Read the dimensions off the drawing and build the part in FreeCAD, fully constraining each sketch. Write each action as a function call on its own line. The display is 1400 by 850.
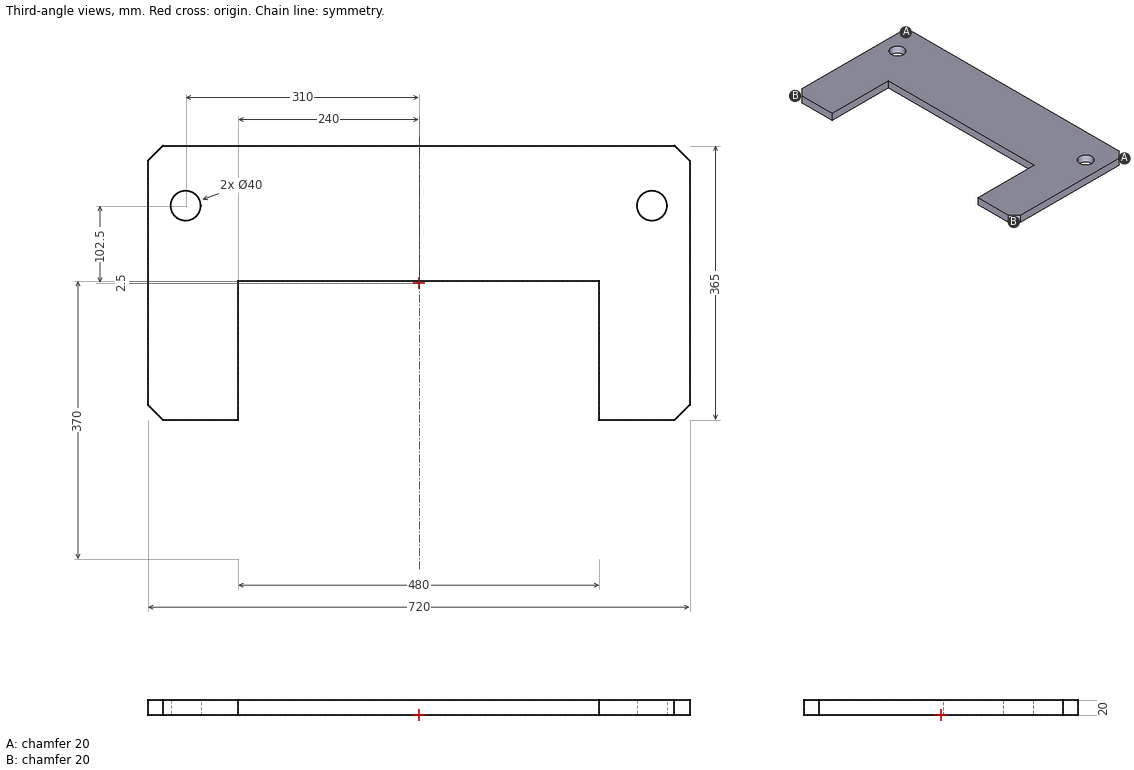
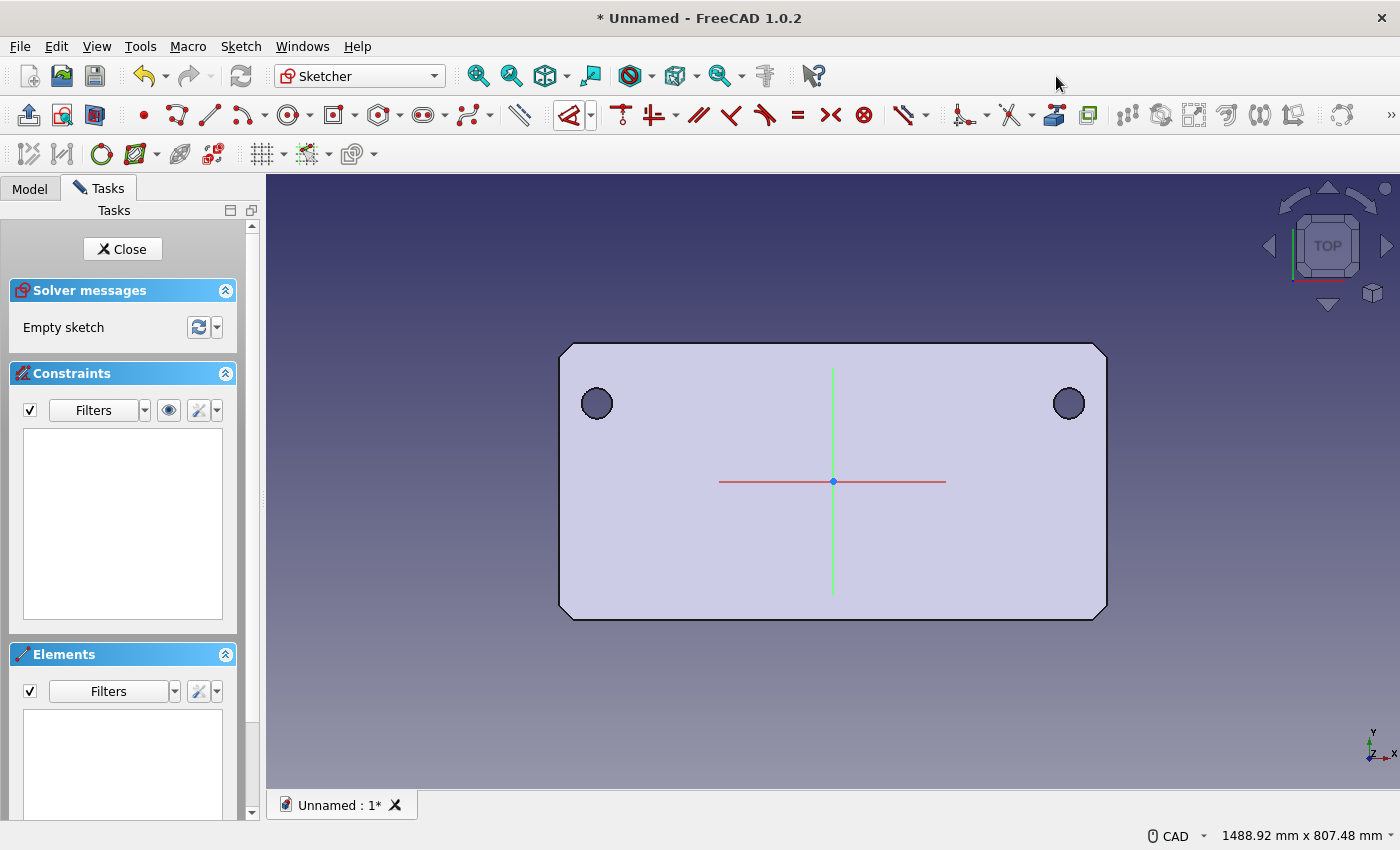
scroll(455, 202, down, 1)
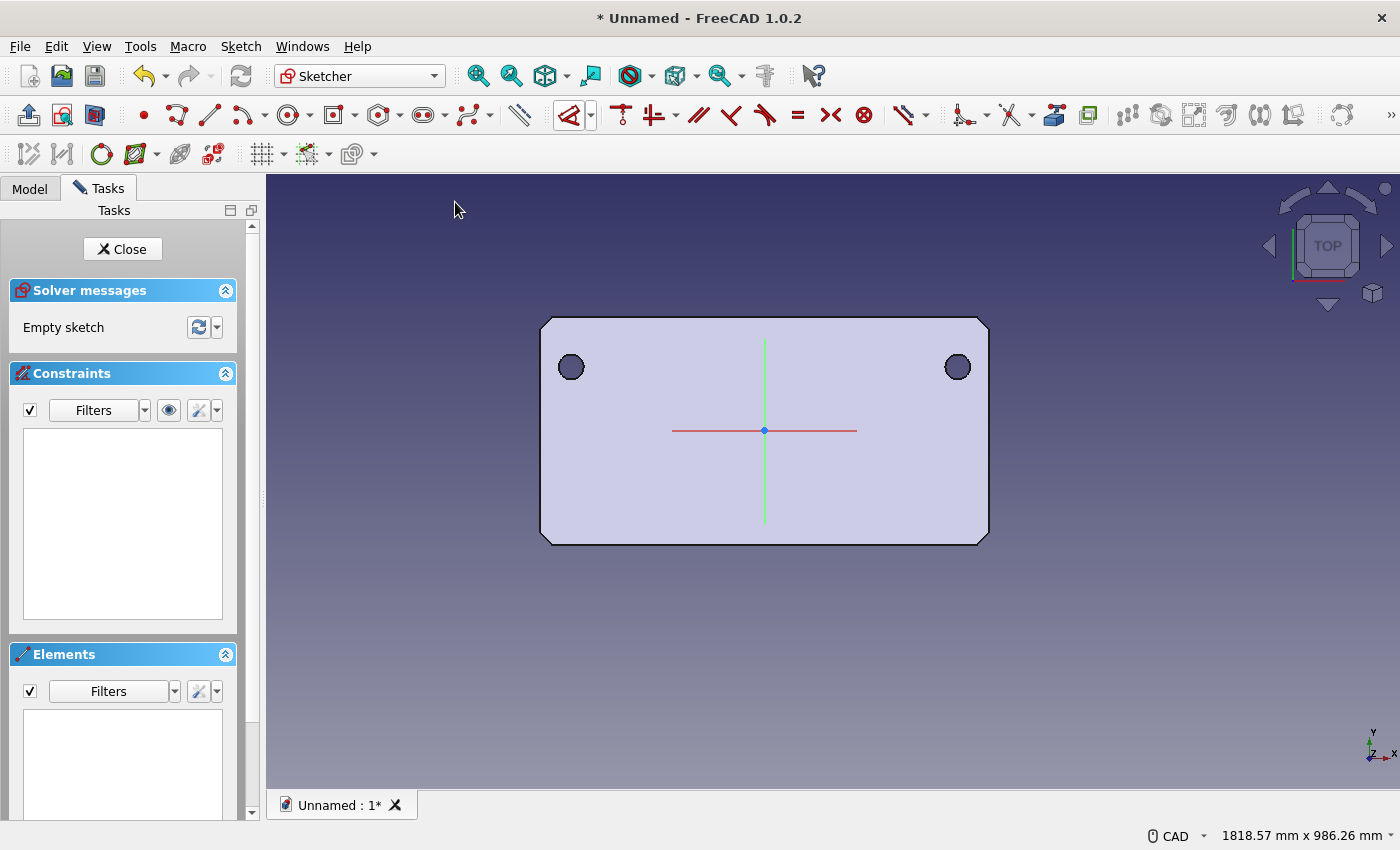
scroll(765, 621, up, 3)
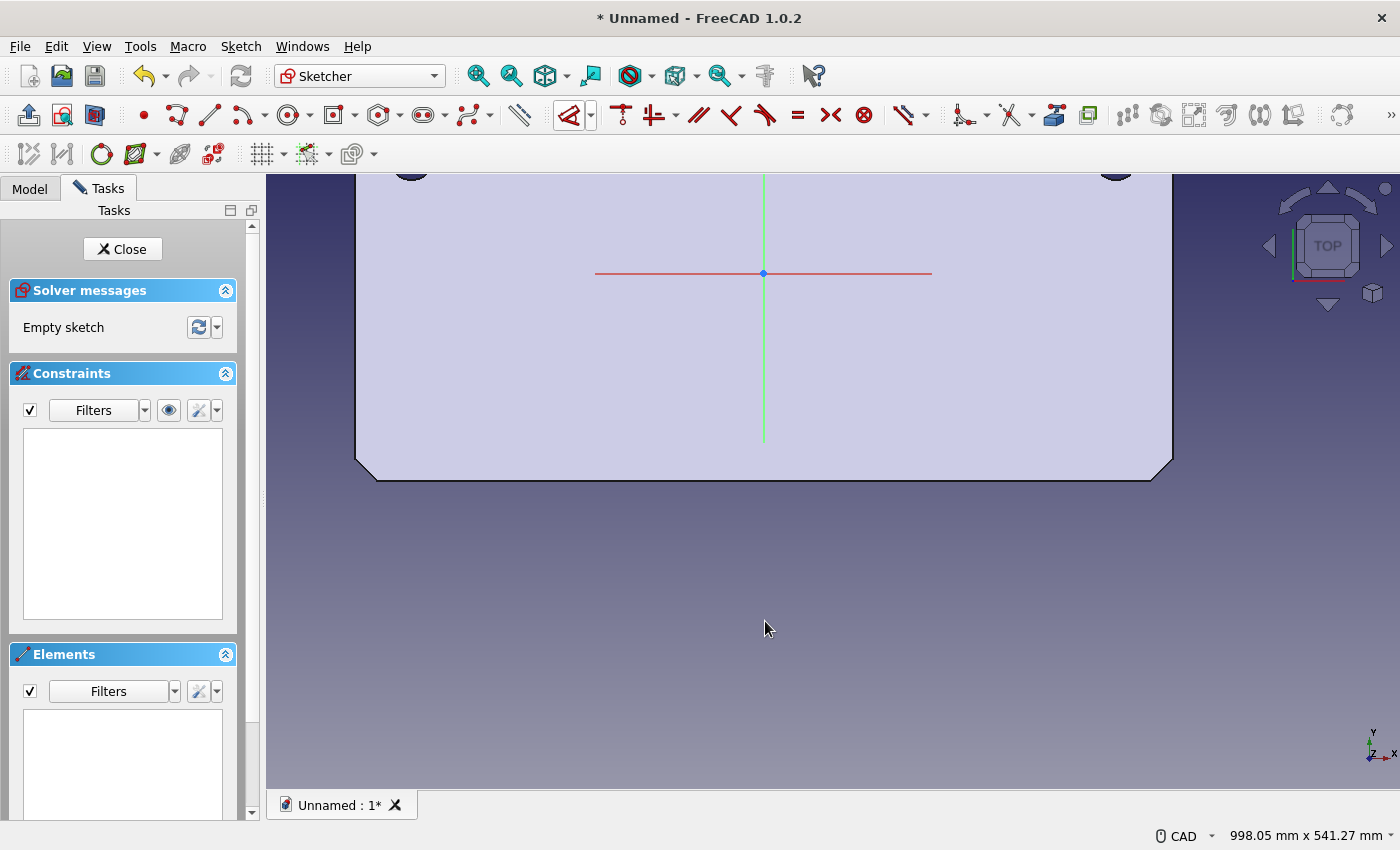
key(g)
key(r)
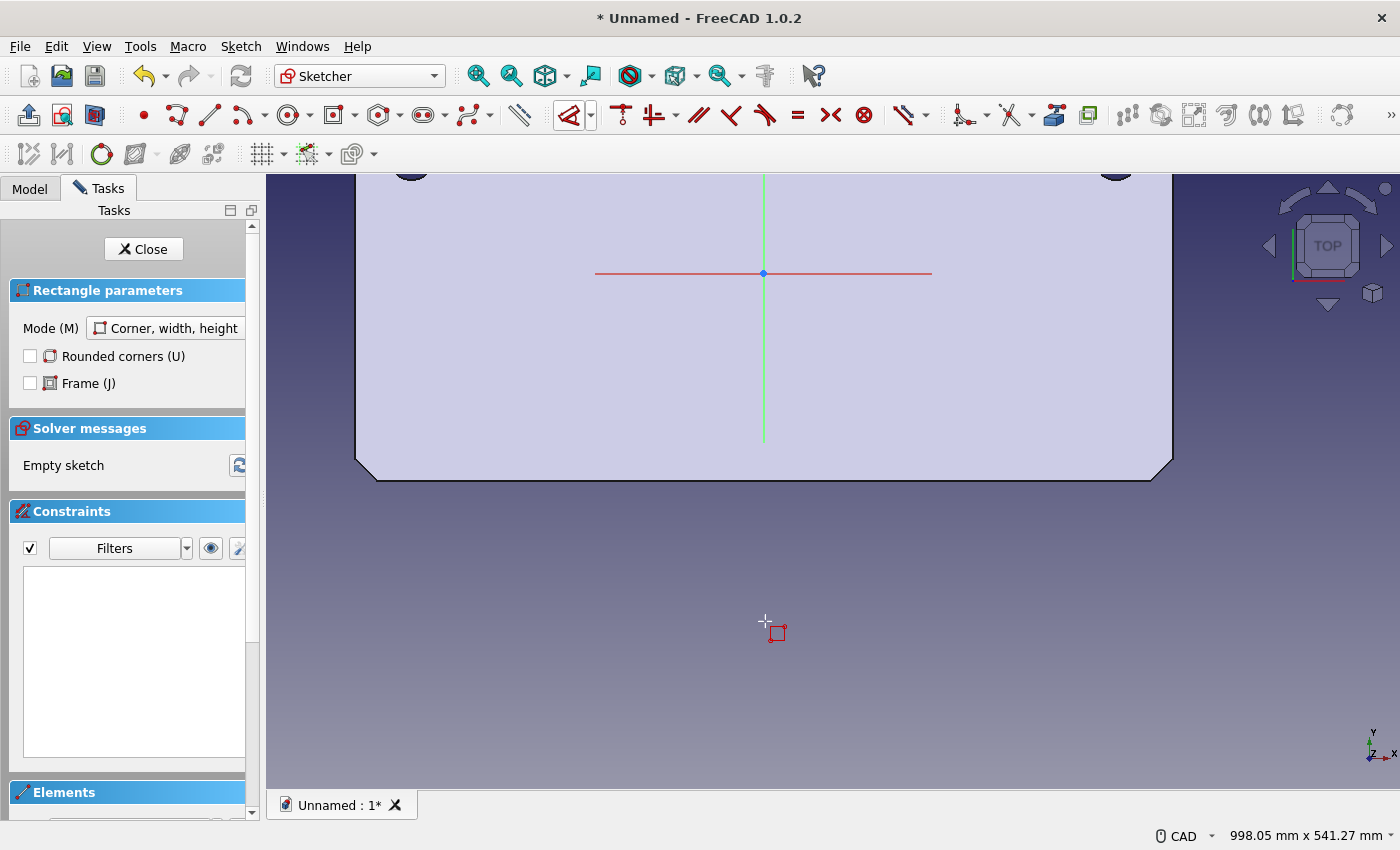
scroll(491, 271, up, 9)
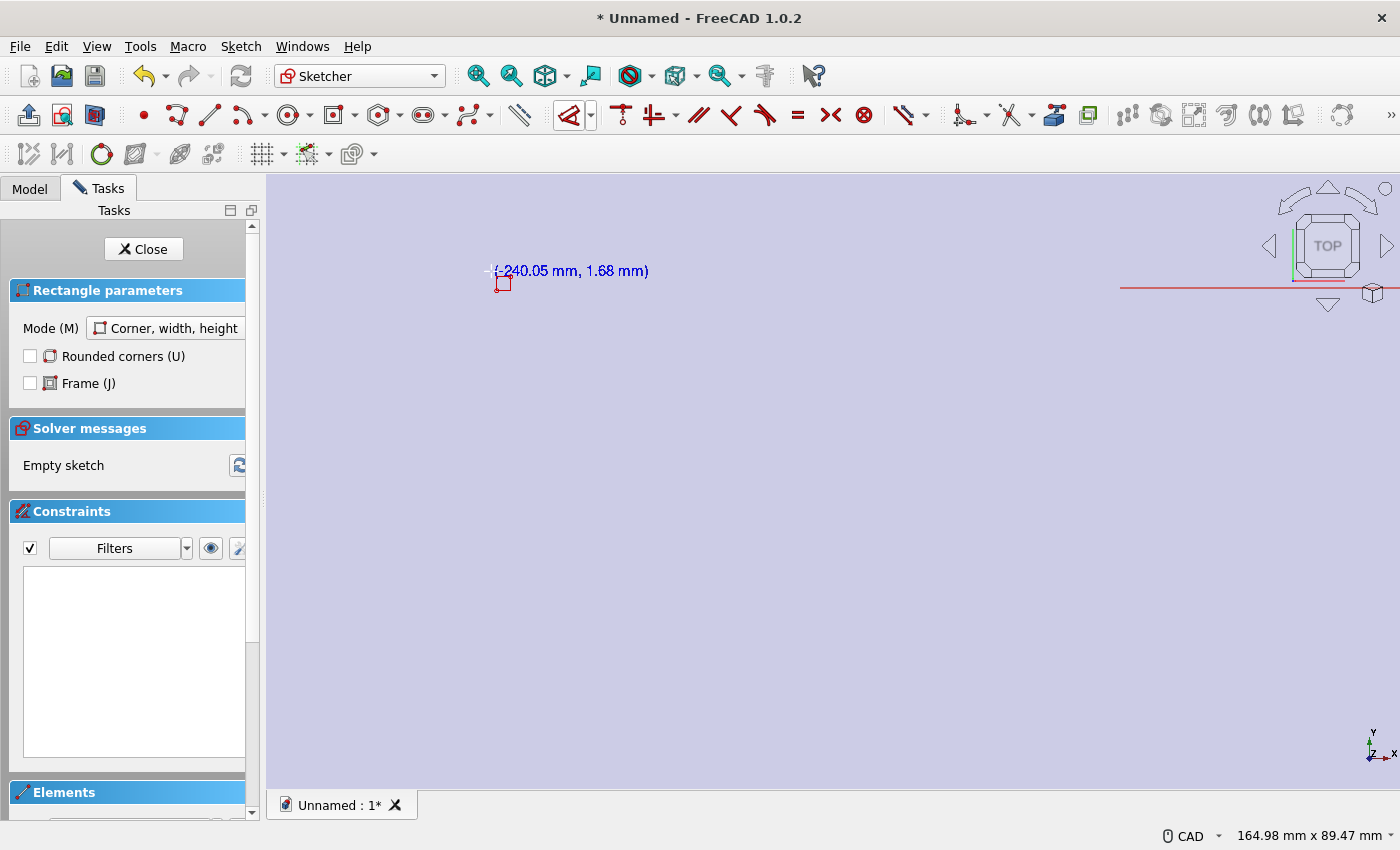
click(490, 271)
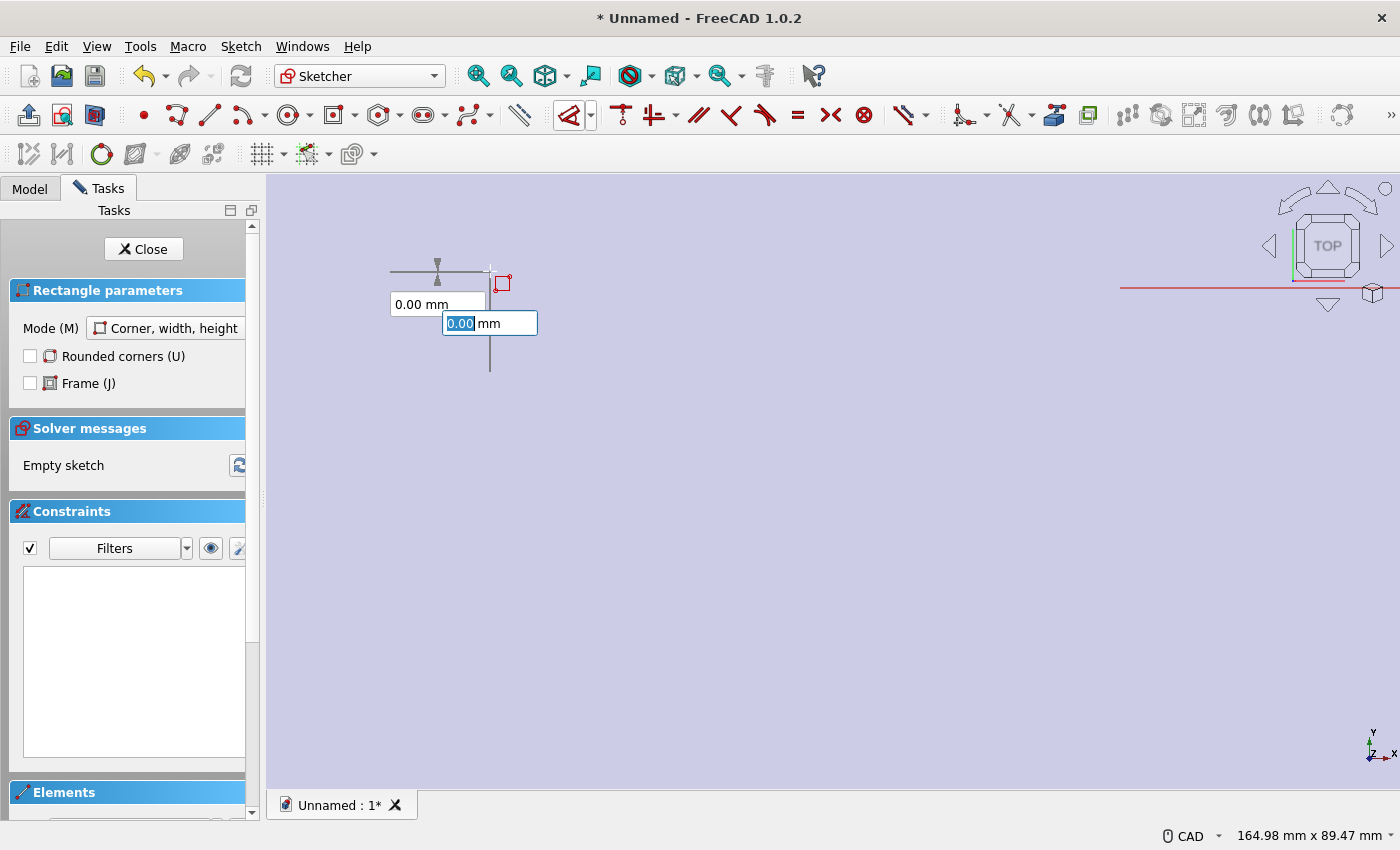
scroll(492, 271, down, 9)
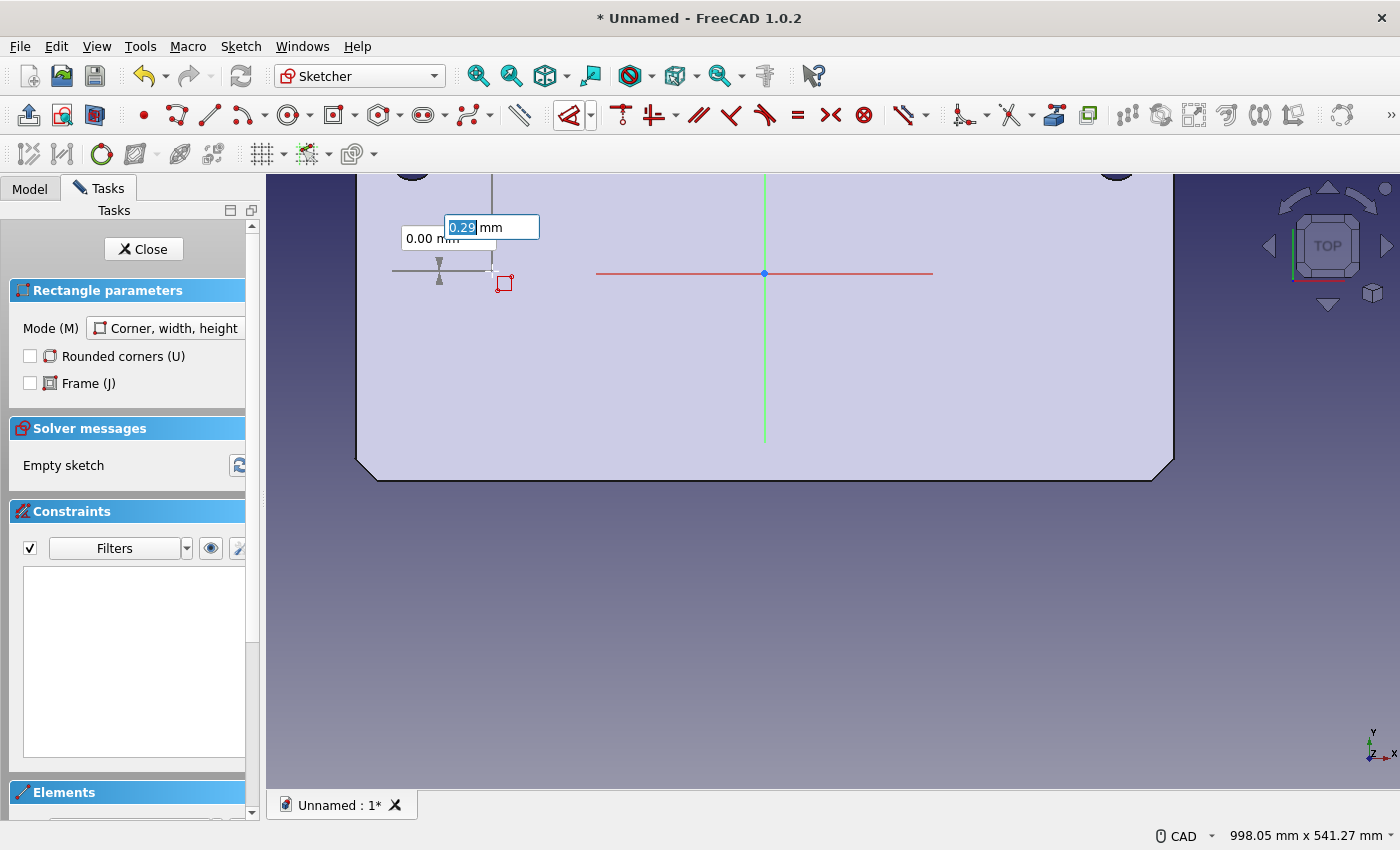
click(1037, 691)
key(Escape)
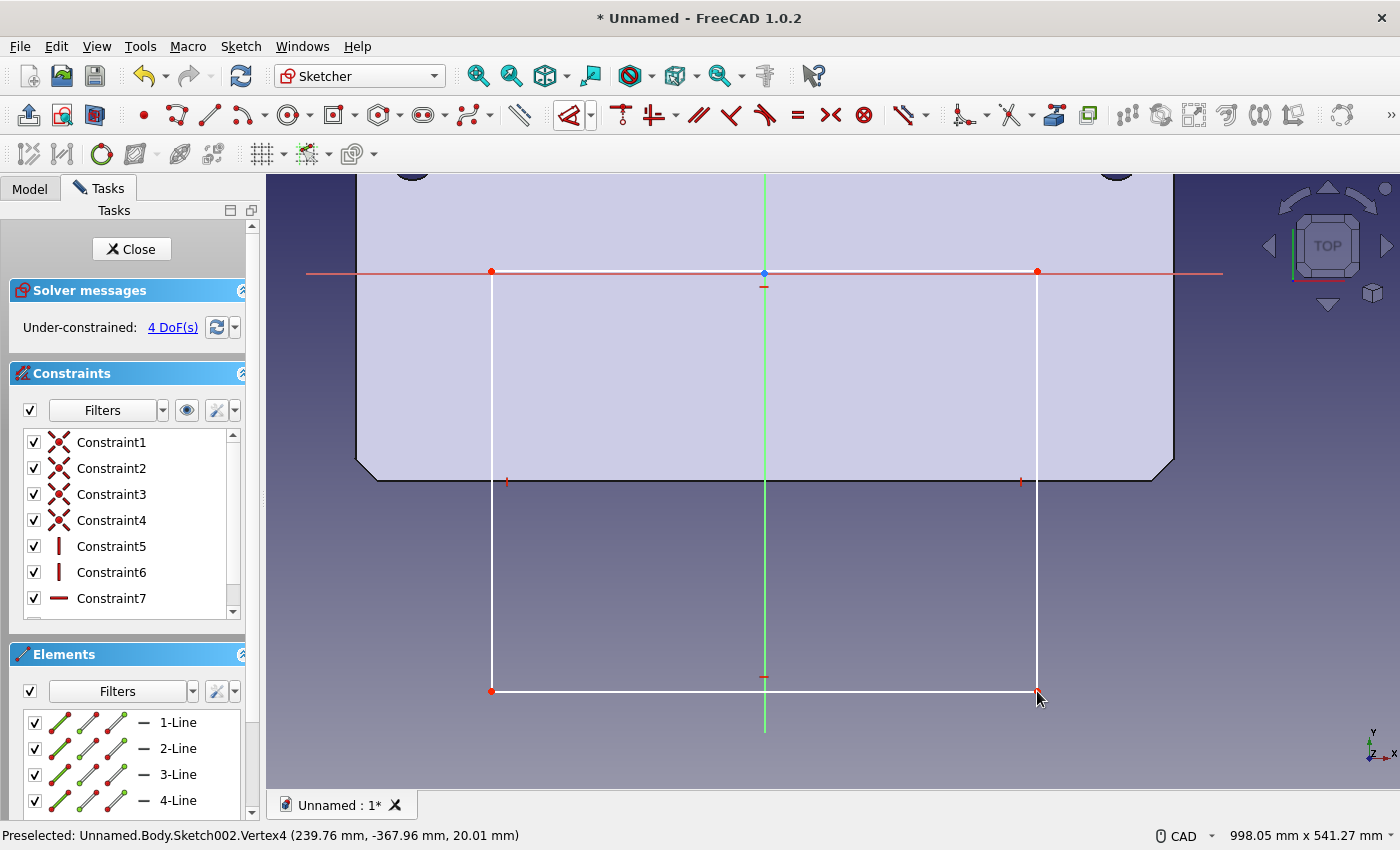
click(492, 398)